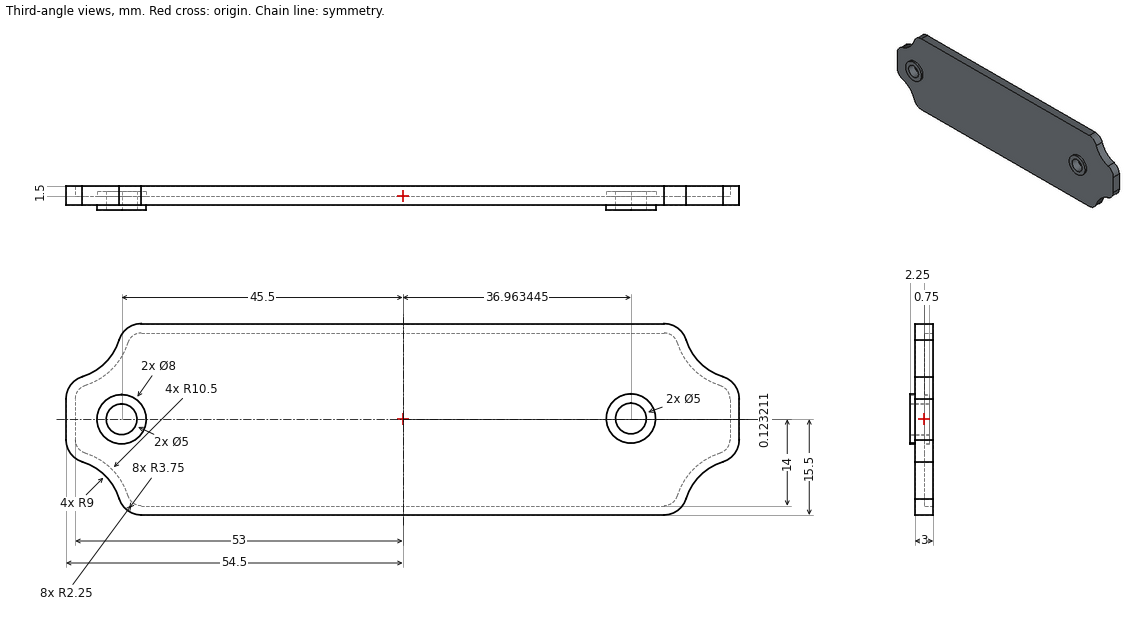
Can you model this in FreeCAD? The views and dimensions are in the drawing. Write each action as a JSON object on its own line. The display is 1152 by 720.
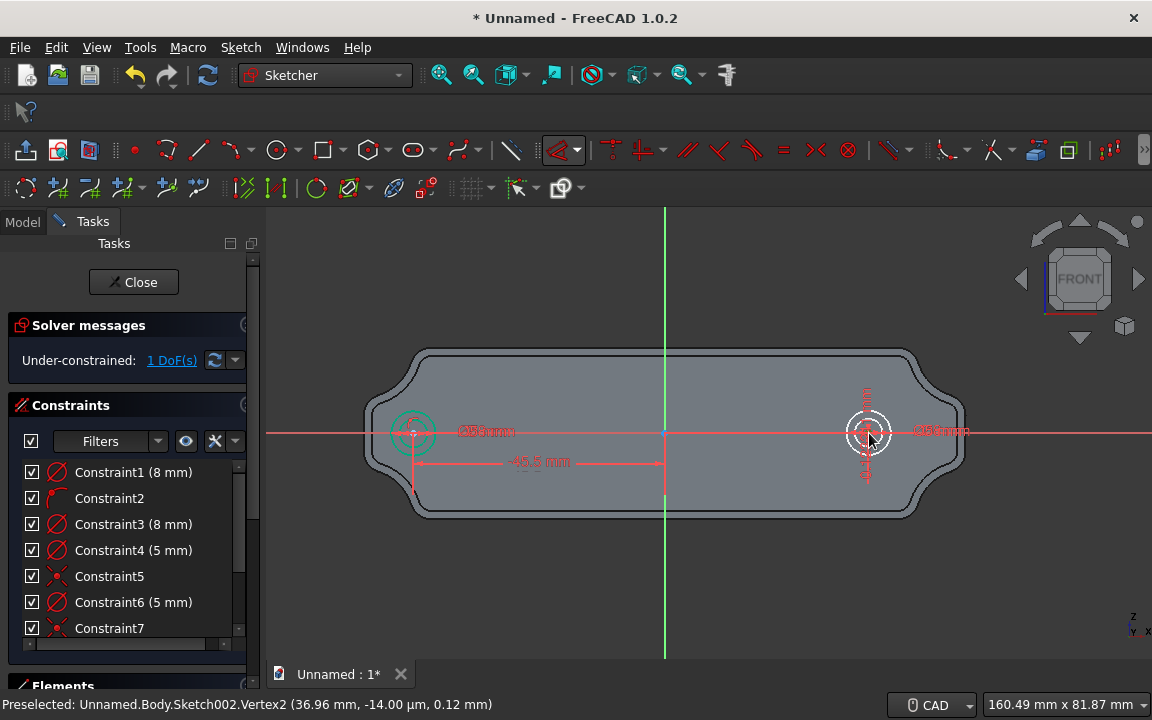
{"action": "left_click", "coordinate": [580, 150]}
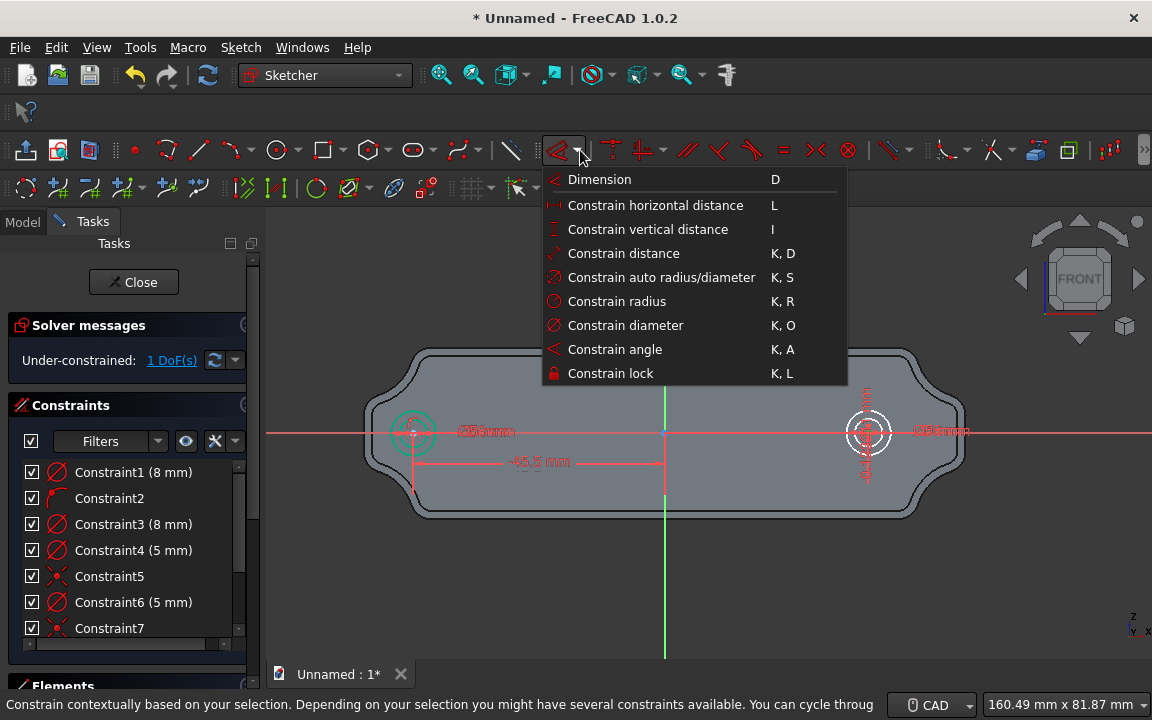
{"action": "left_click", "coordinate": [695, 205]}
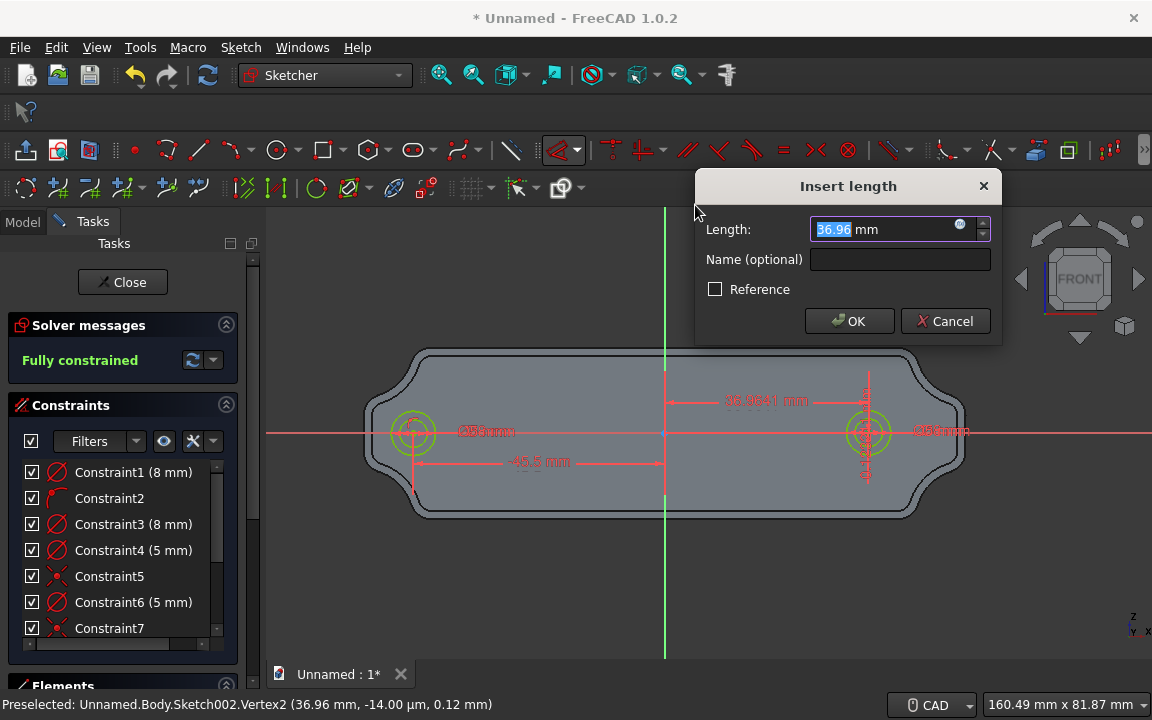
{"action": "type", "text": "36.963445"}
{"action": "key", "text": "Return"}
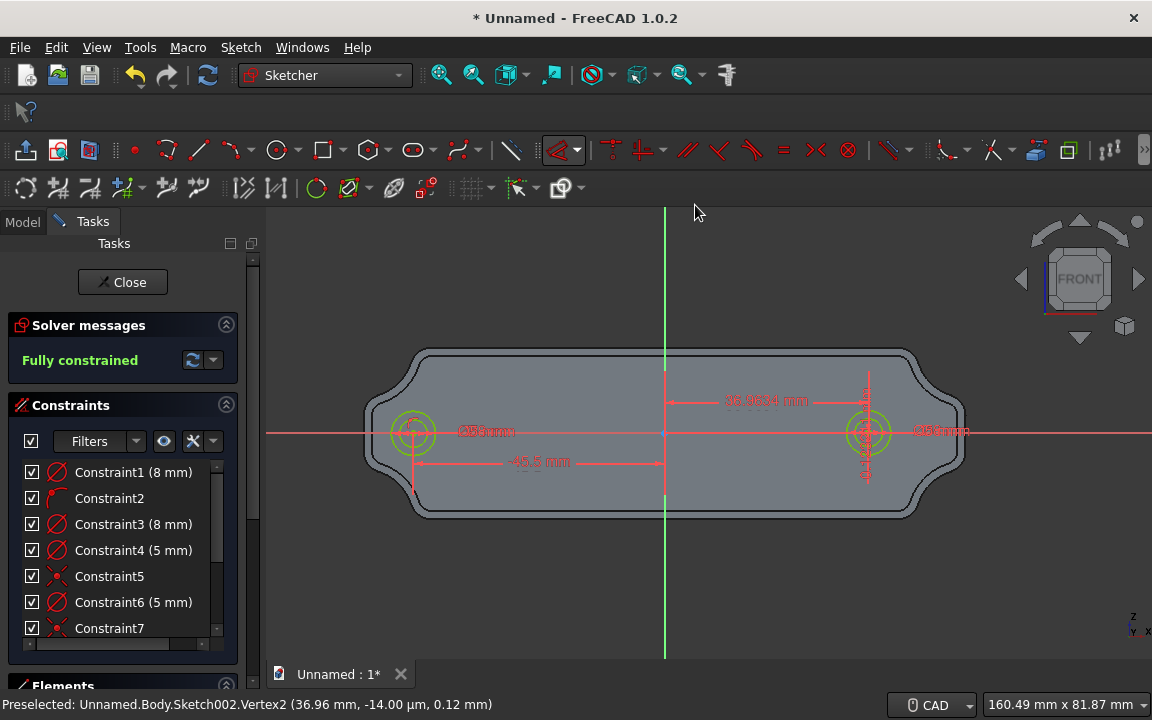
{"action": "left_click", "coordinate": [123, 282]}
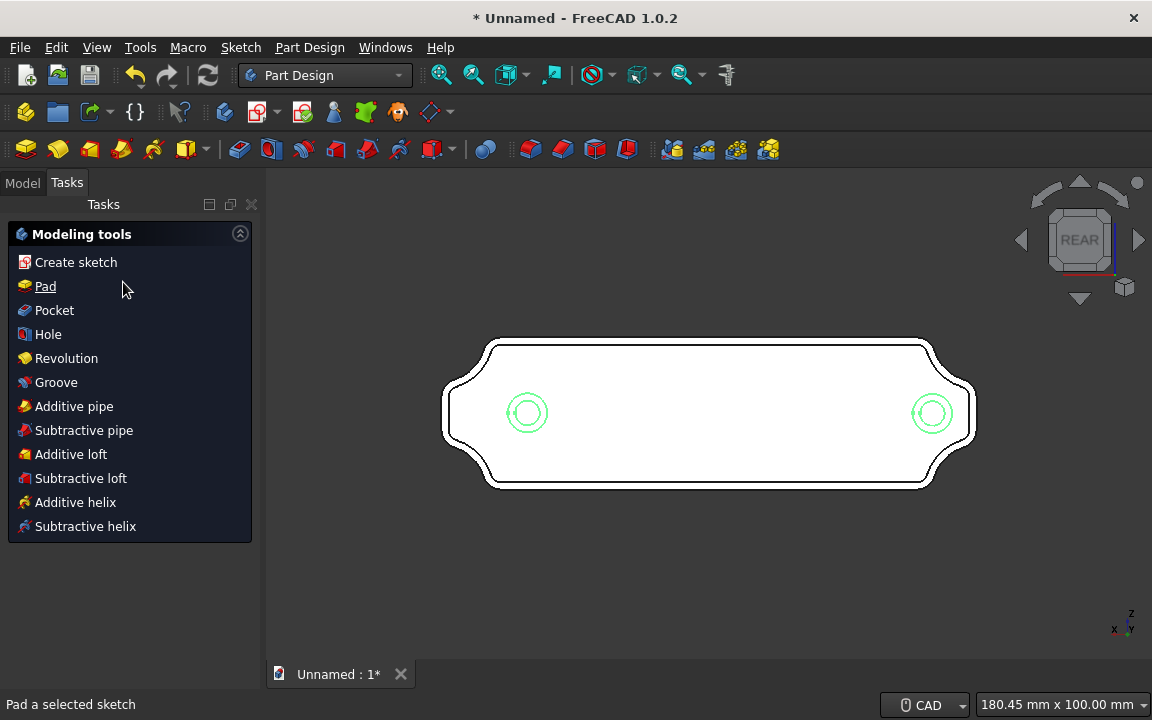
{"action": "left_click", "coordinate": [26, 150]}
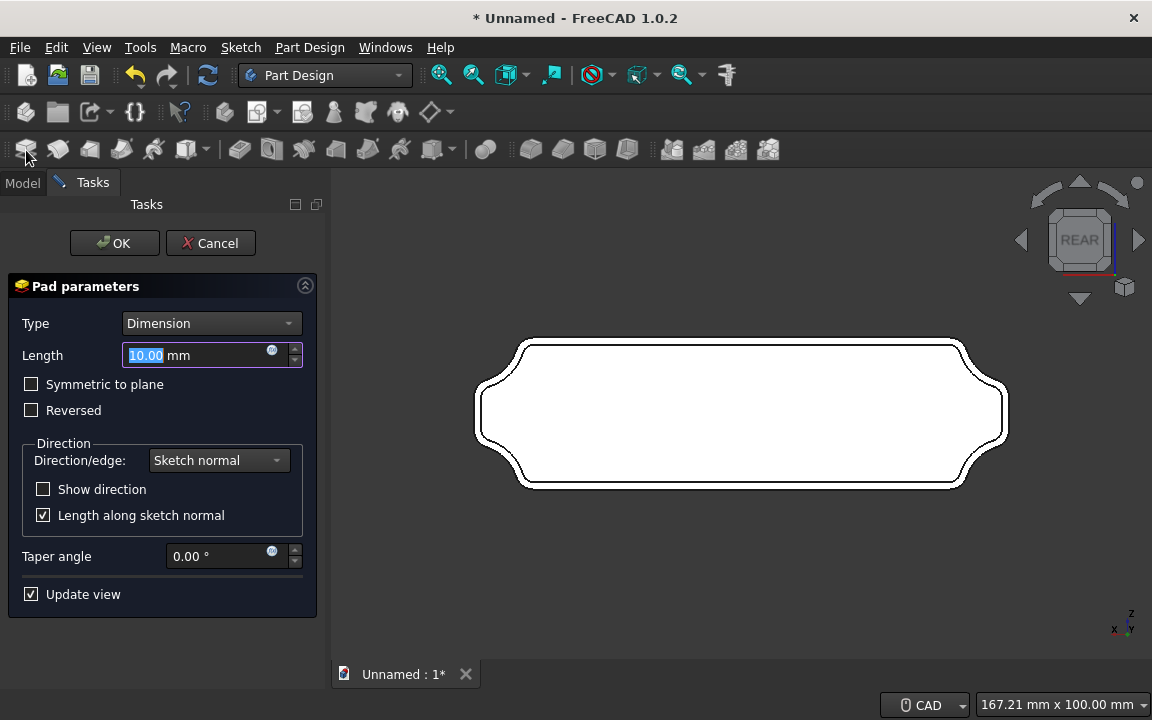
{"action": "left_click", "coordinate": [212, 324]}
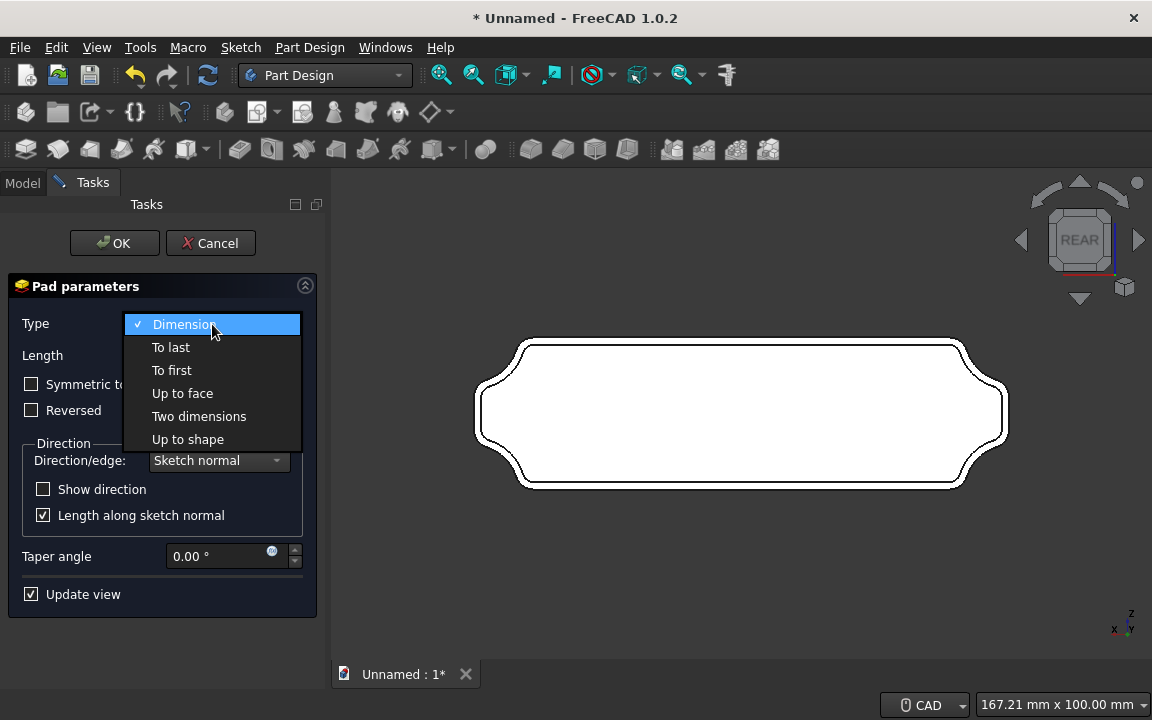
{"action": "left_click", "coordinate": [212, 416]}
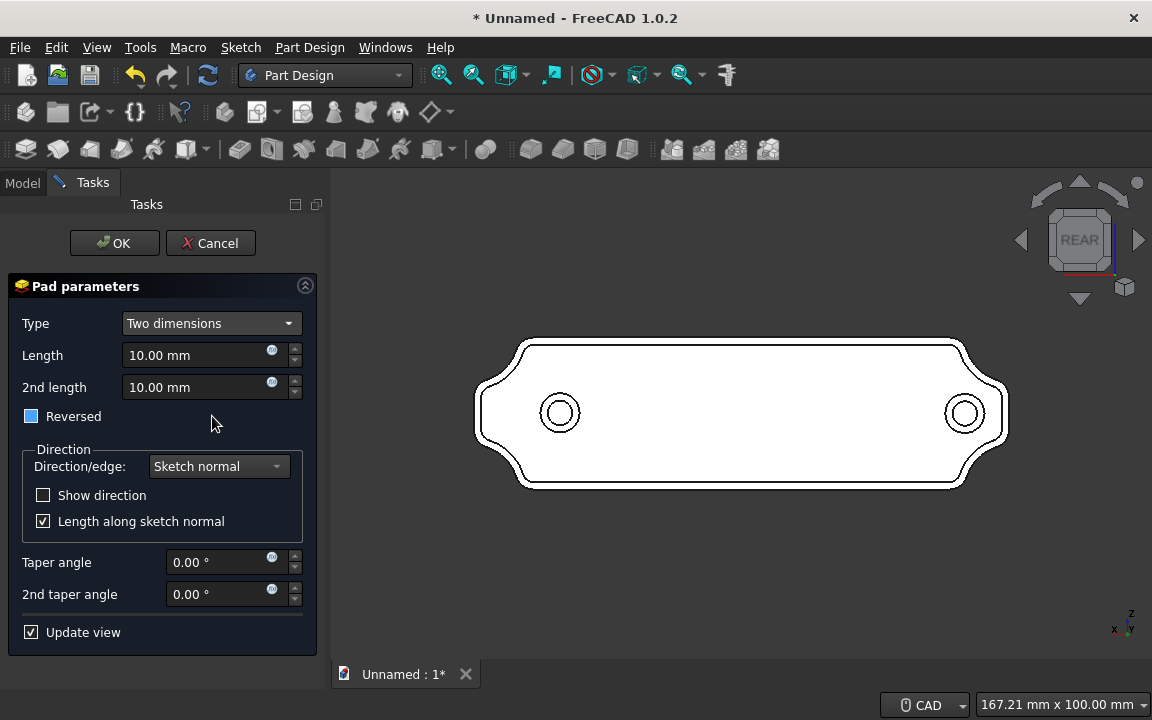
{"action": "triple_click", "coordinate": [204, 355]}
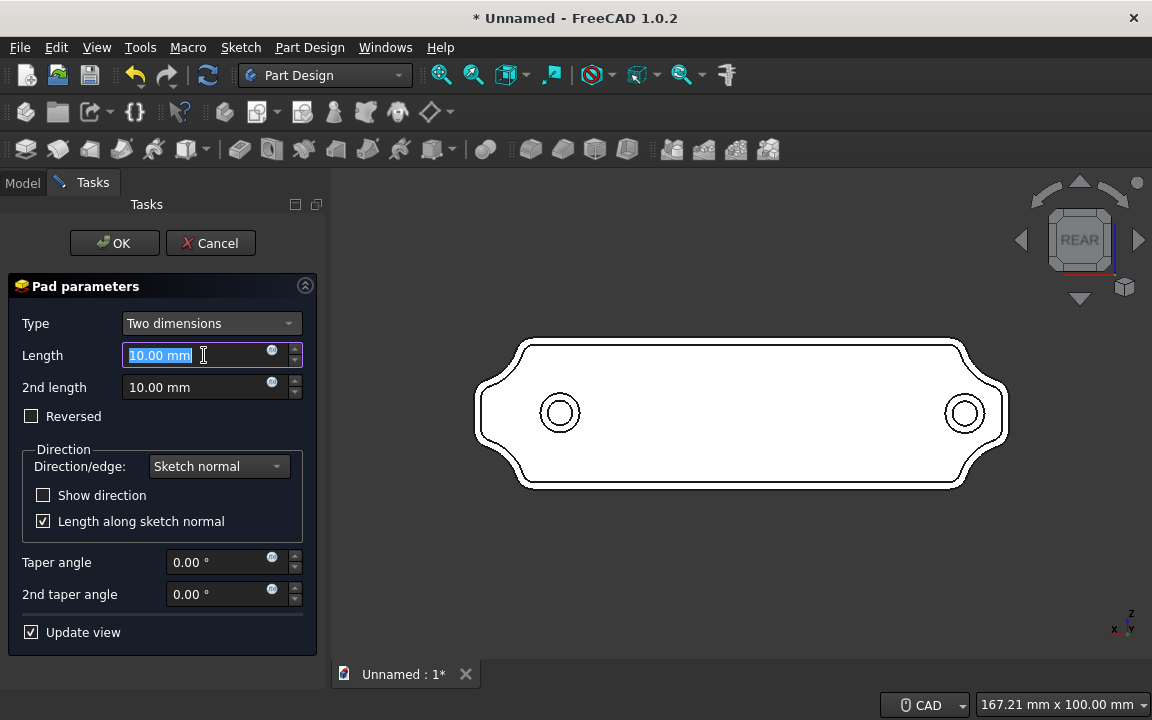
{"action": "type", "text": "0.75"}
{"action": "key", "text": "Tab"}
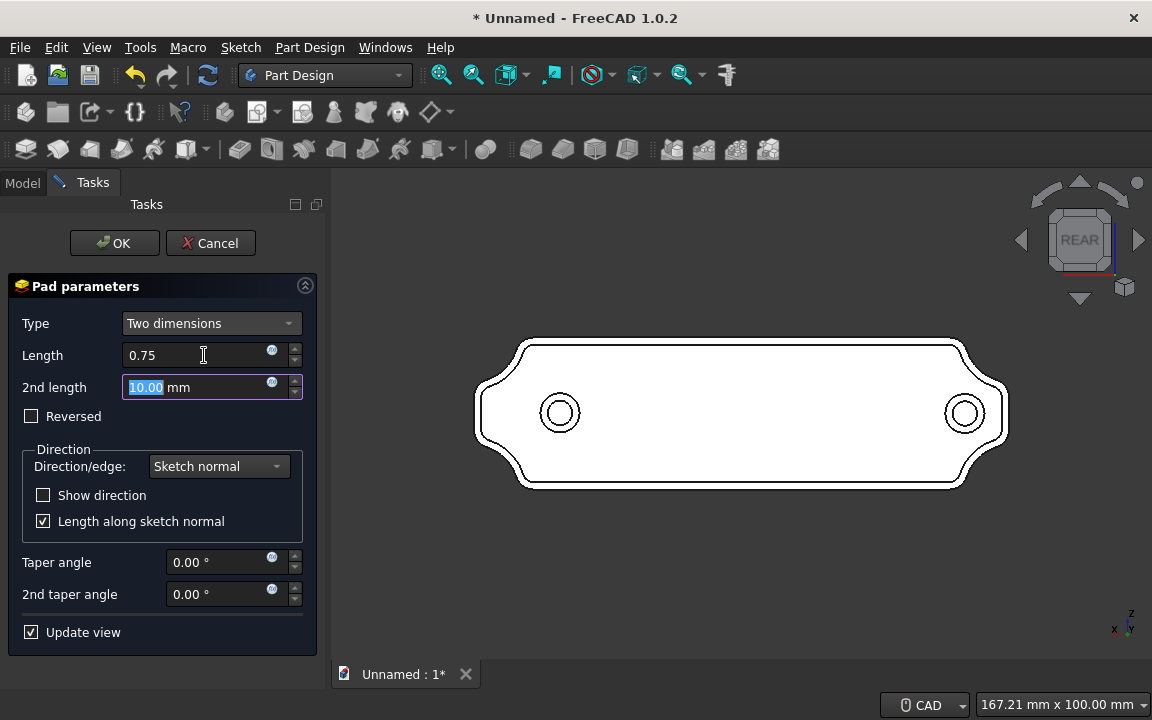
{"action": "type", "text": "2.25"}
{"action": "key", "text": "Tab"}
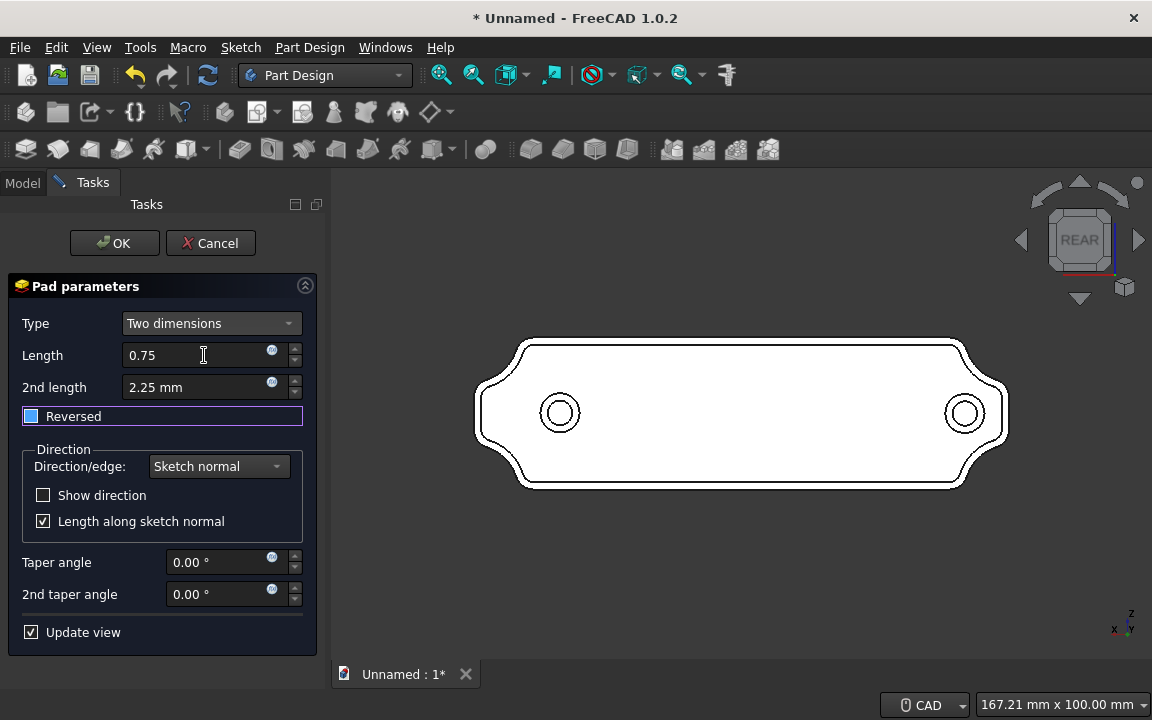
{"action": "left_click", "coordinate": [30, 416]}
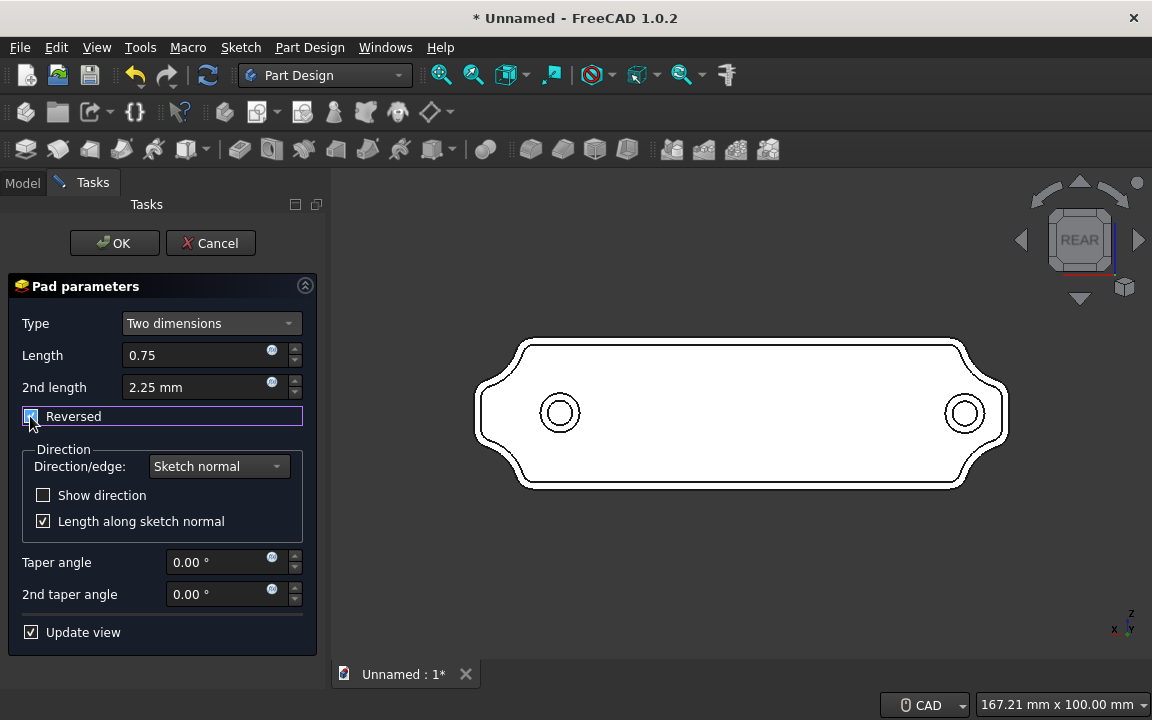
{"action": "left_click", "coordinate": [115, 243]}